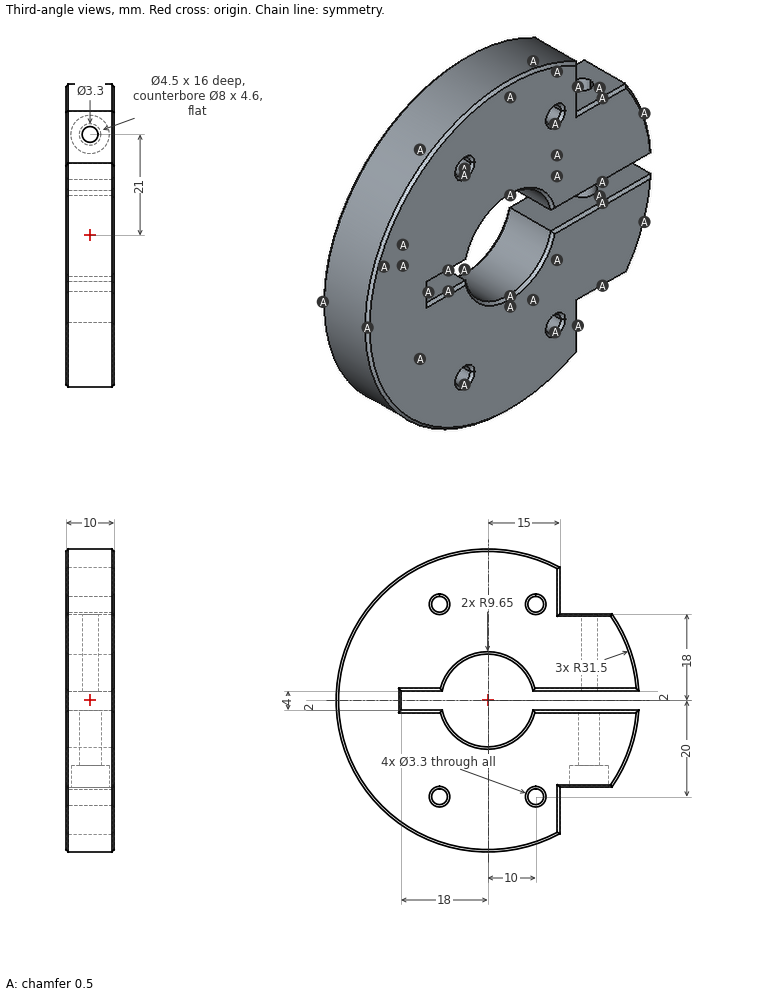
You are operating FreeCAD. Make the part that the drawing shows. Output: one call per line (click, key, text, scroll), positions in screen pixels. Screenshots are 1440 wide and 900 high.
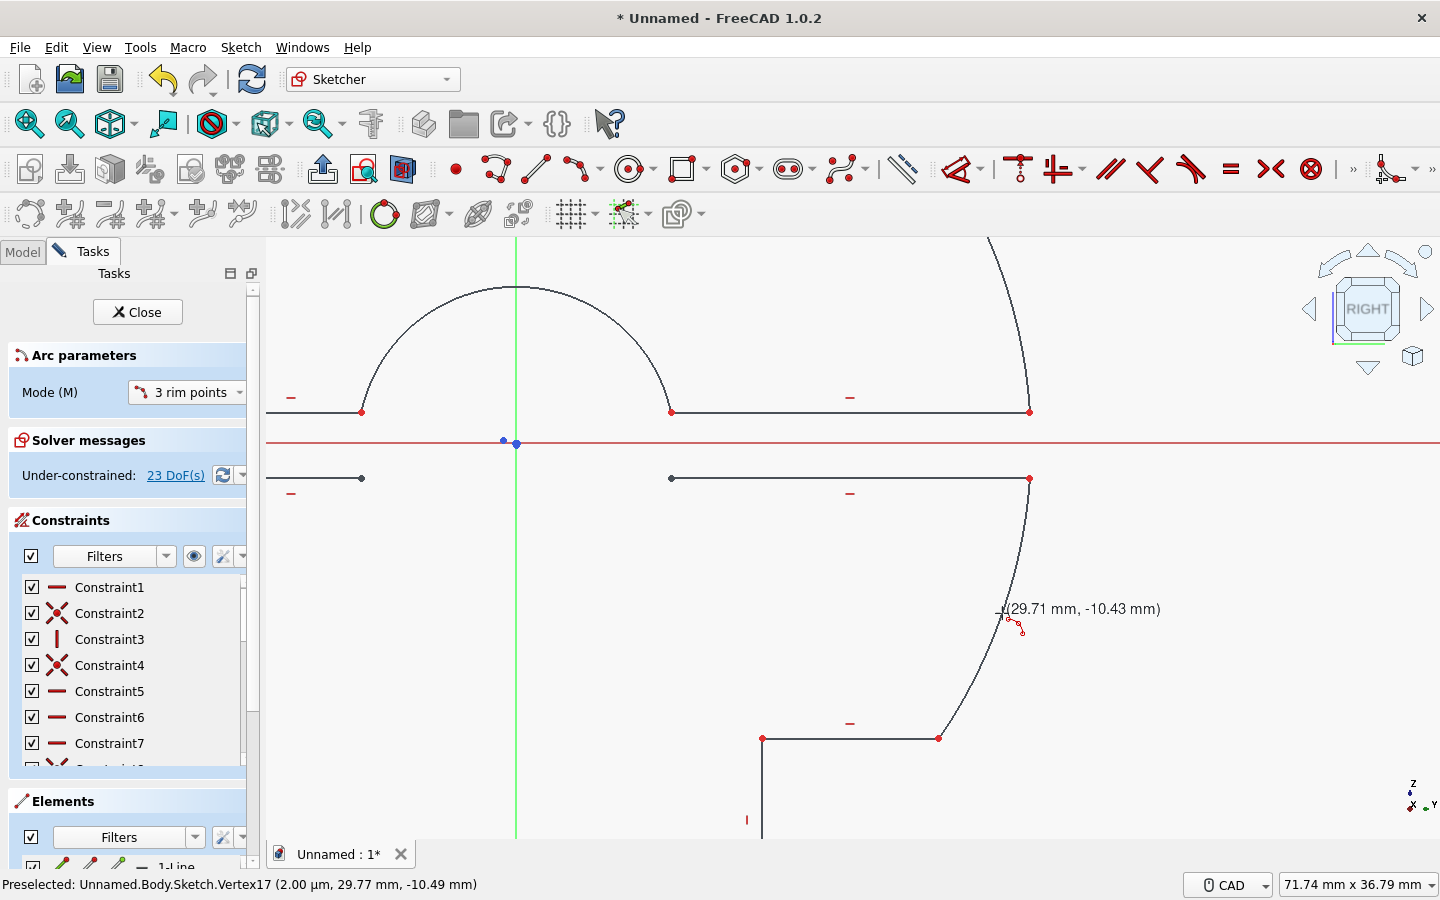
click(671, 478)
click(361, 478)
click(473, 595)
key(Escape)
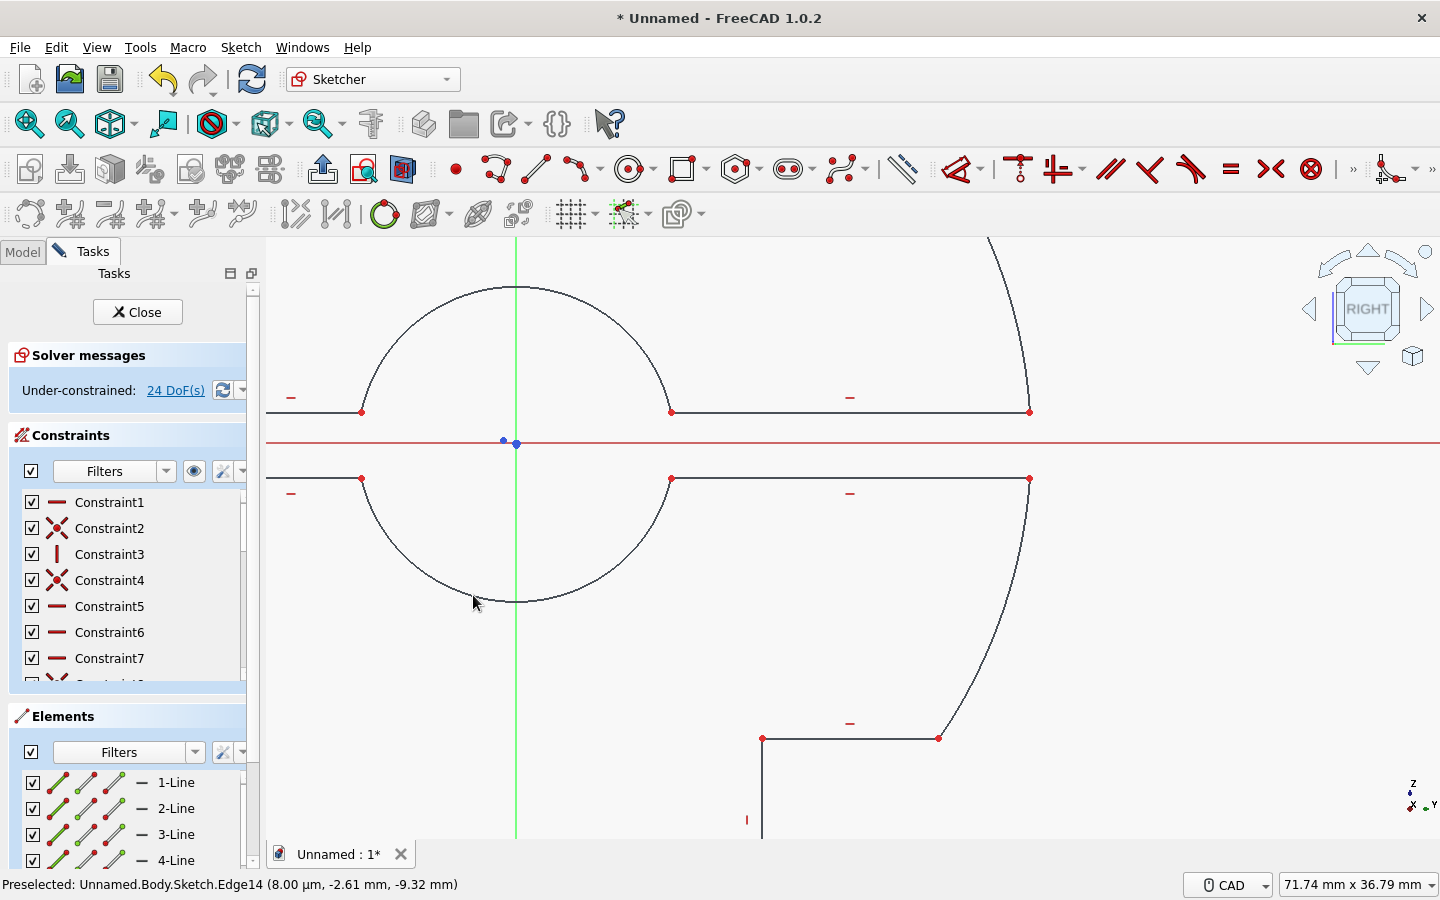
click(598, 310)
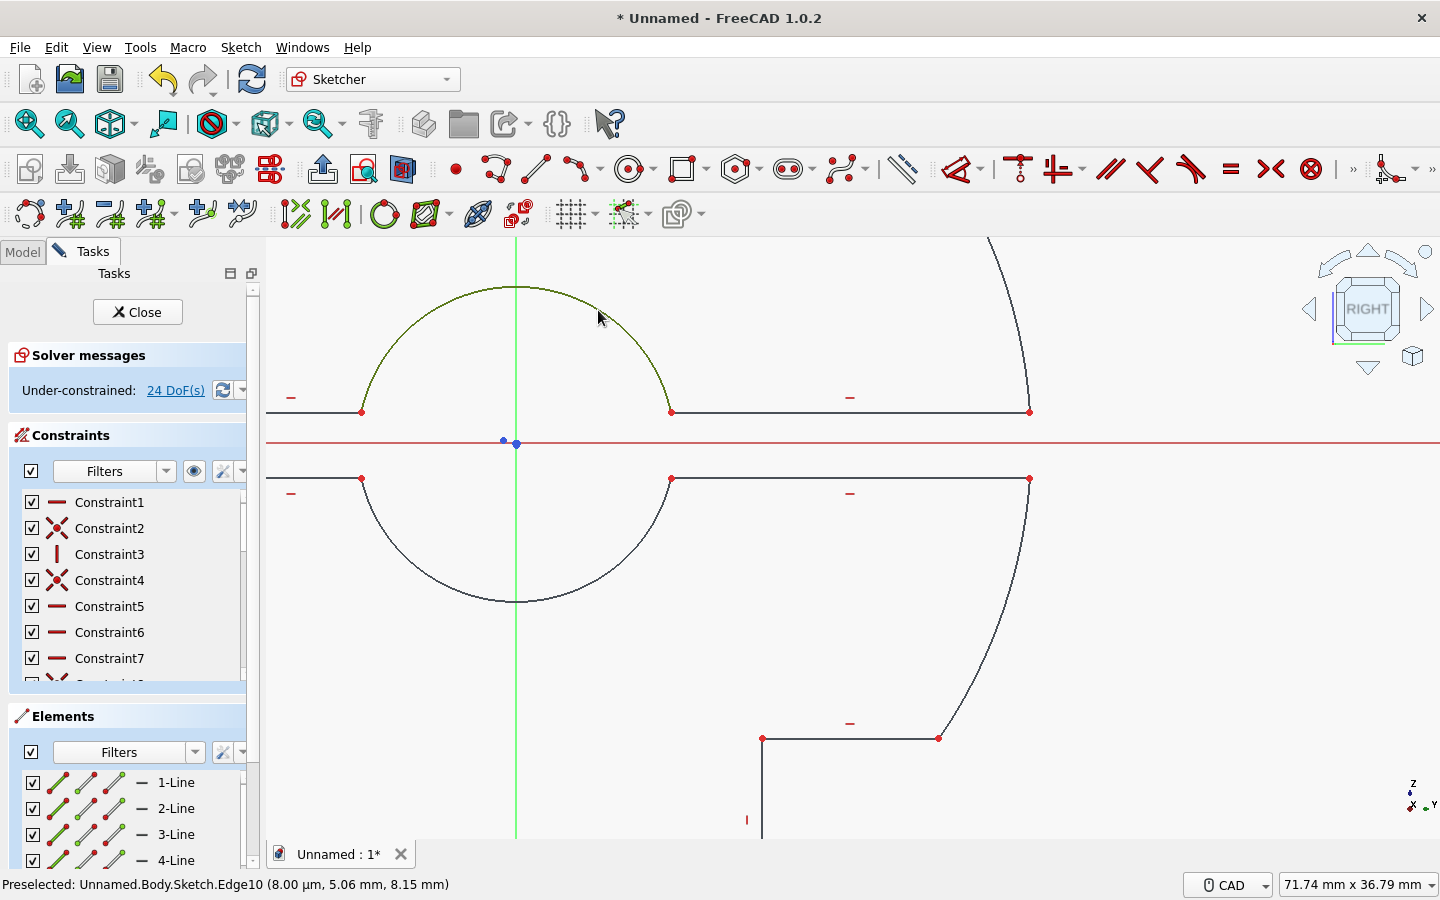
click(1018, 329)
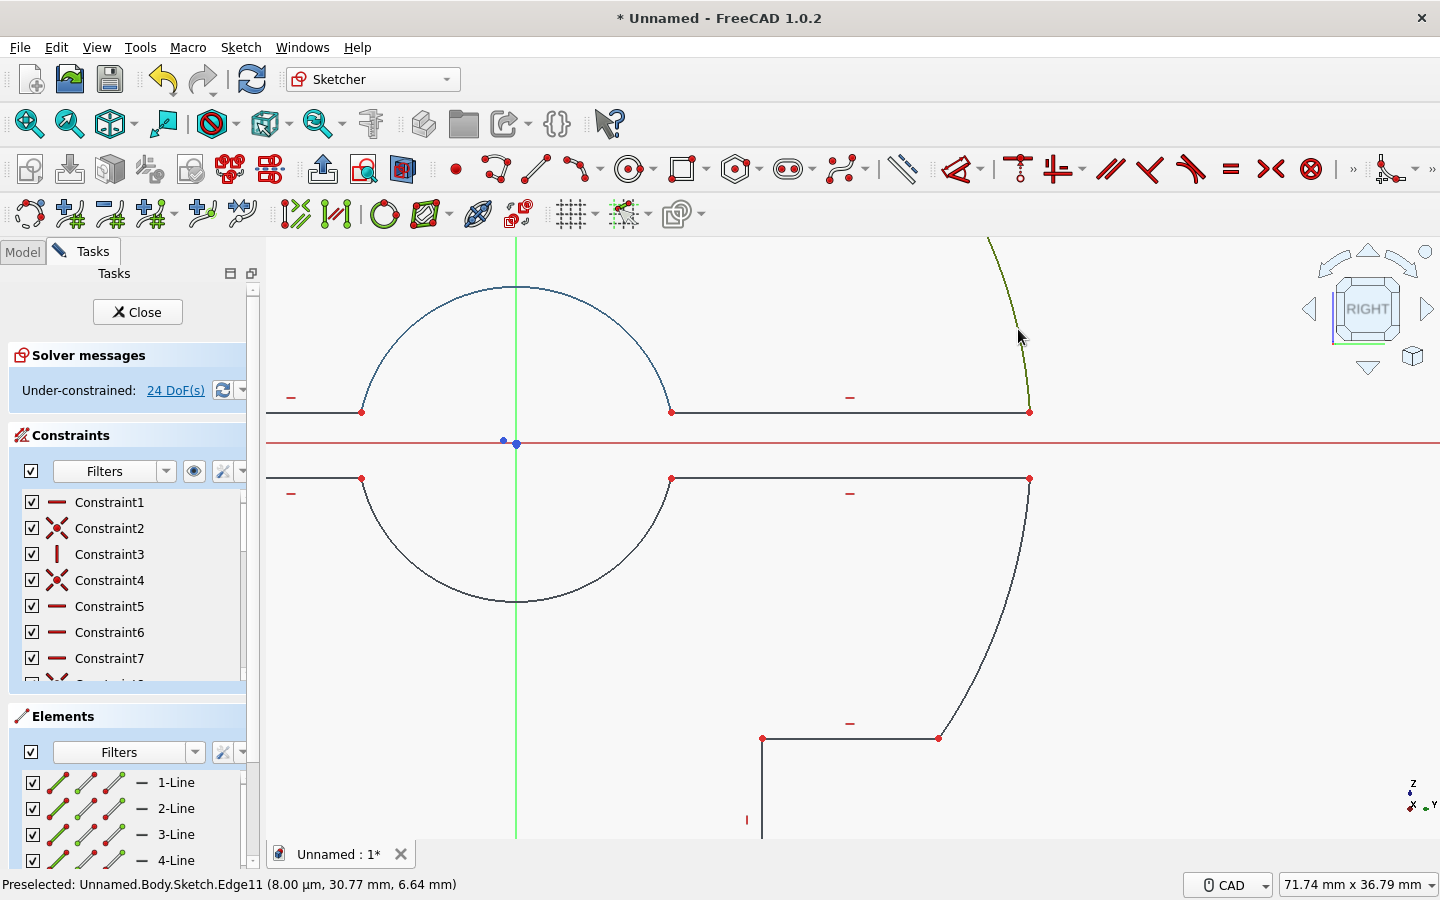
key(c)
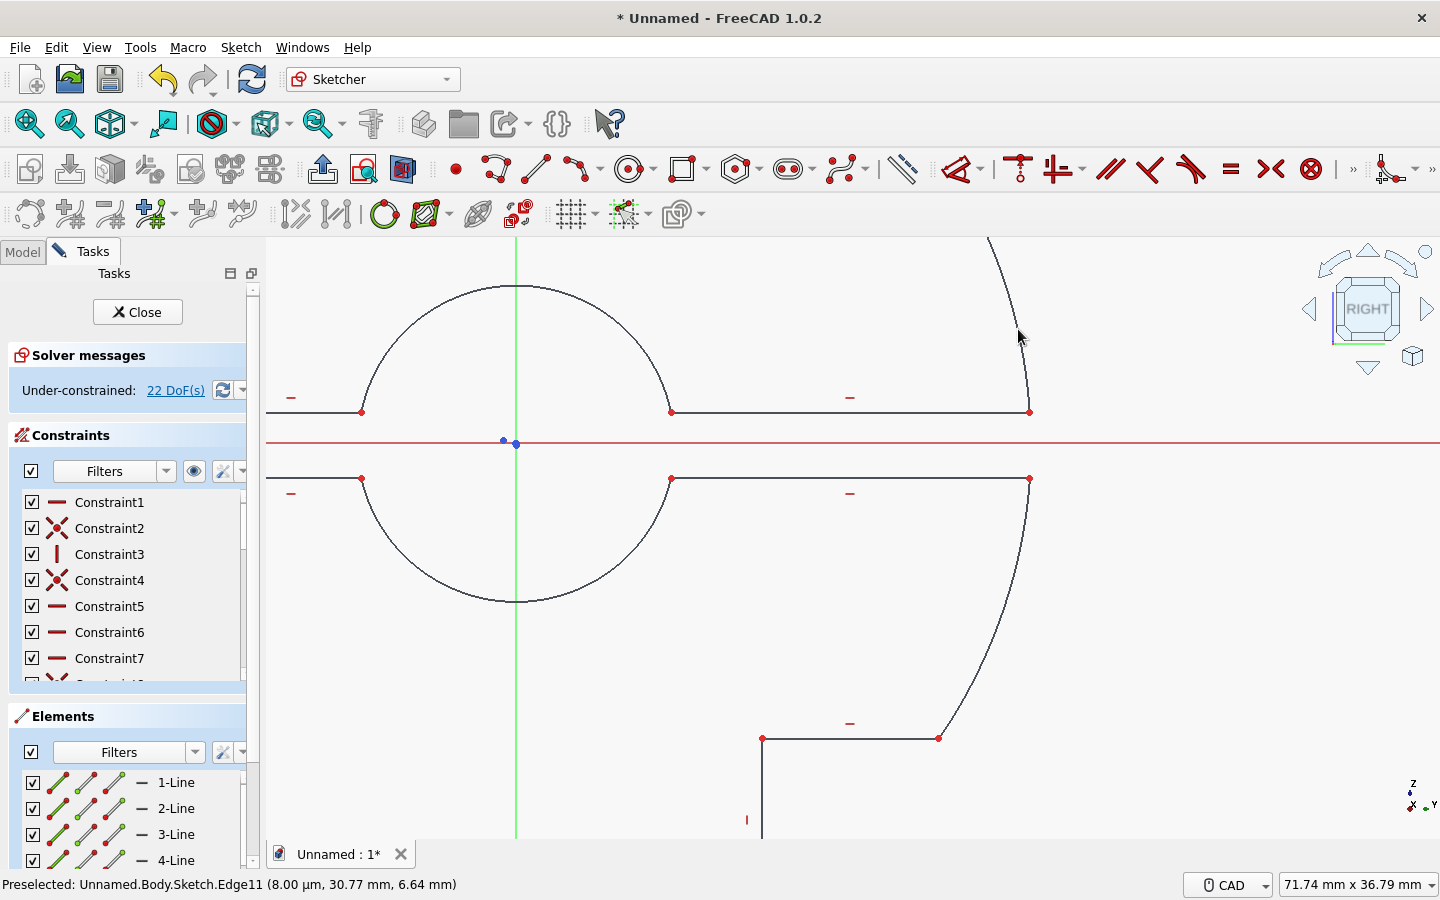
click(599, 309)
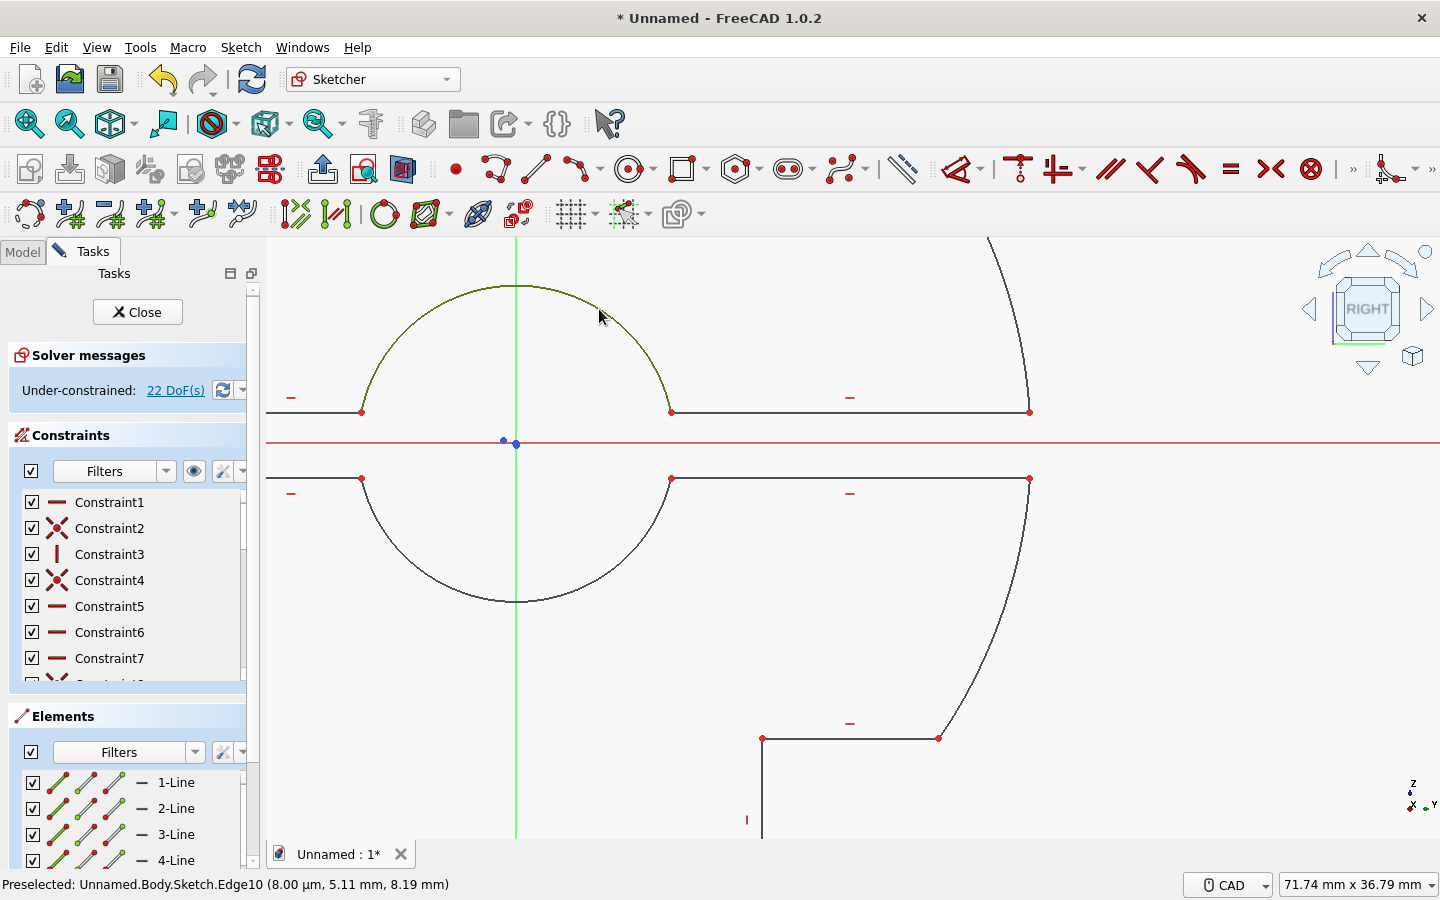
scroll(1004, 615, down, 4)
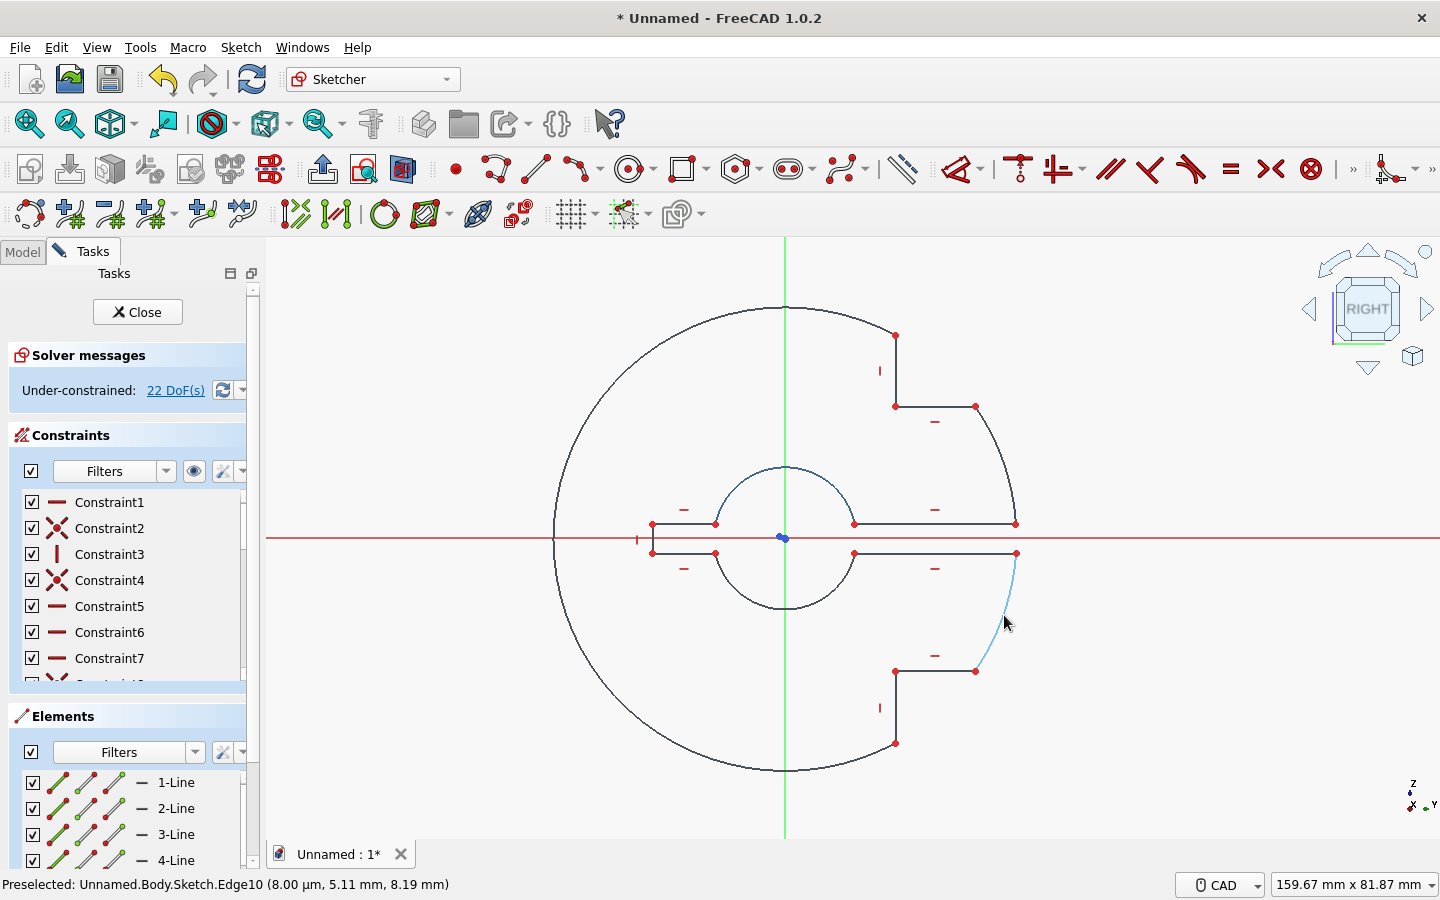
click(628, 369)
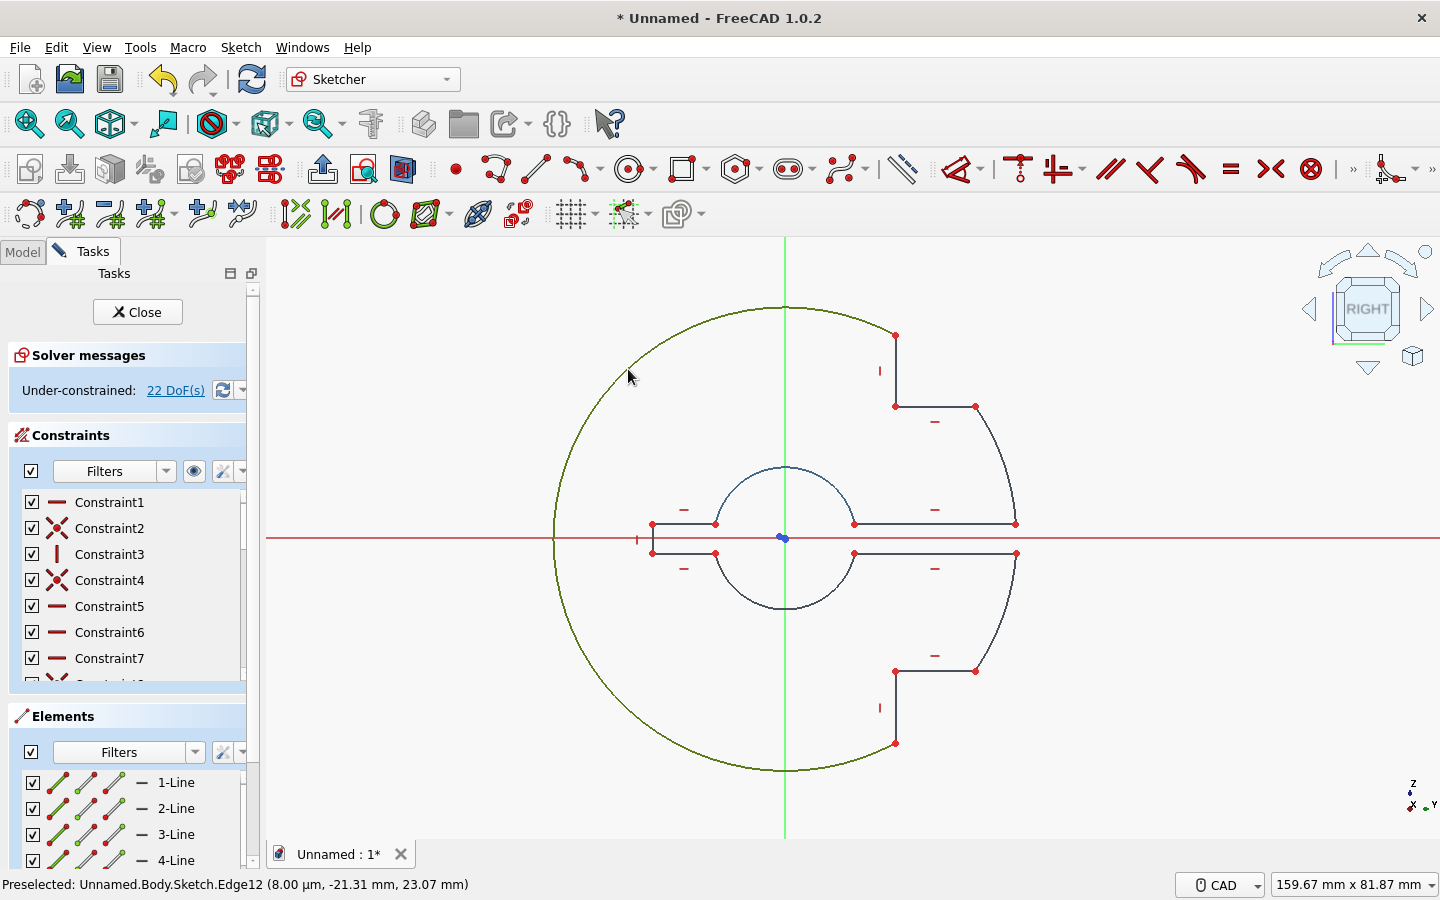
click(1018, 170)